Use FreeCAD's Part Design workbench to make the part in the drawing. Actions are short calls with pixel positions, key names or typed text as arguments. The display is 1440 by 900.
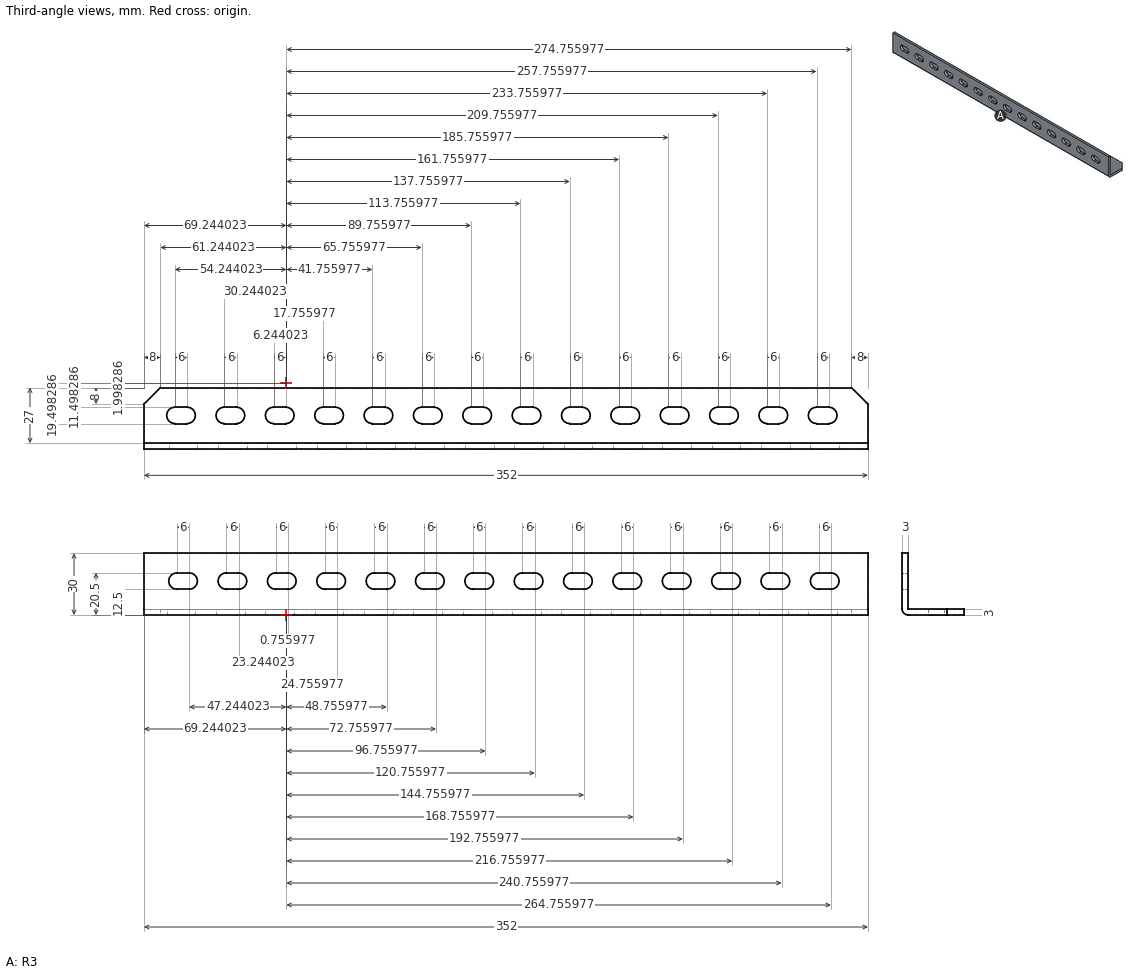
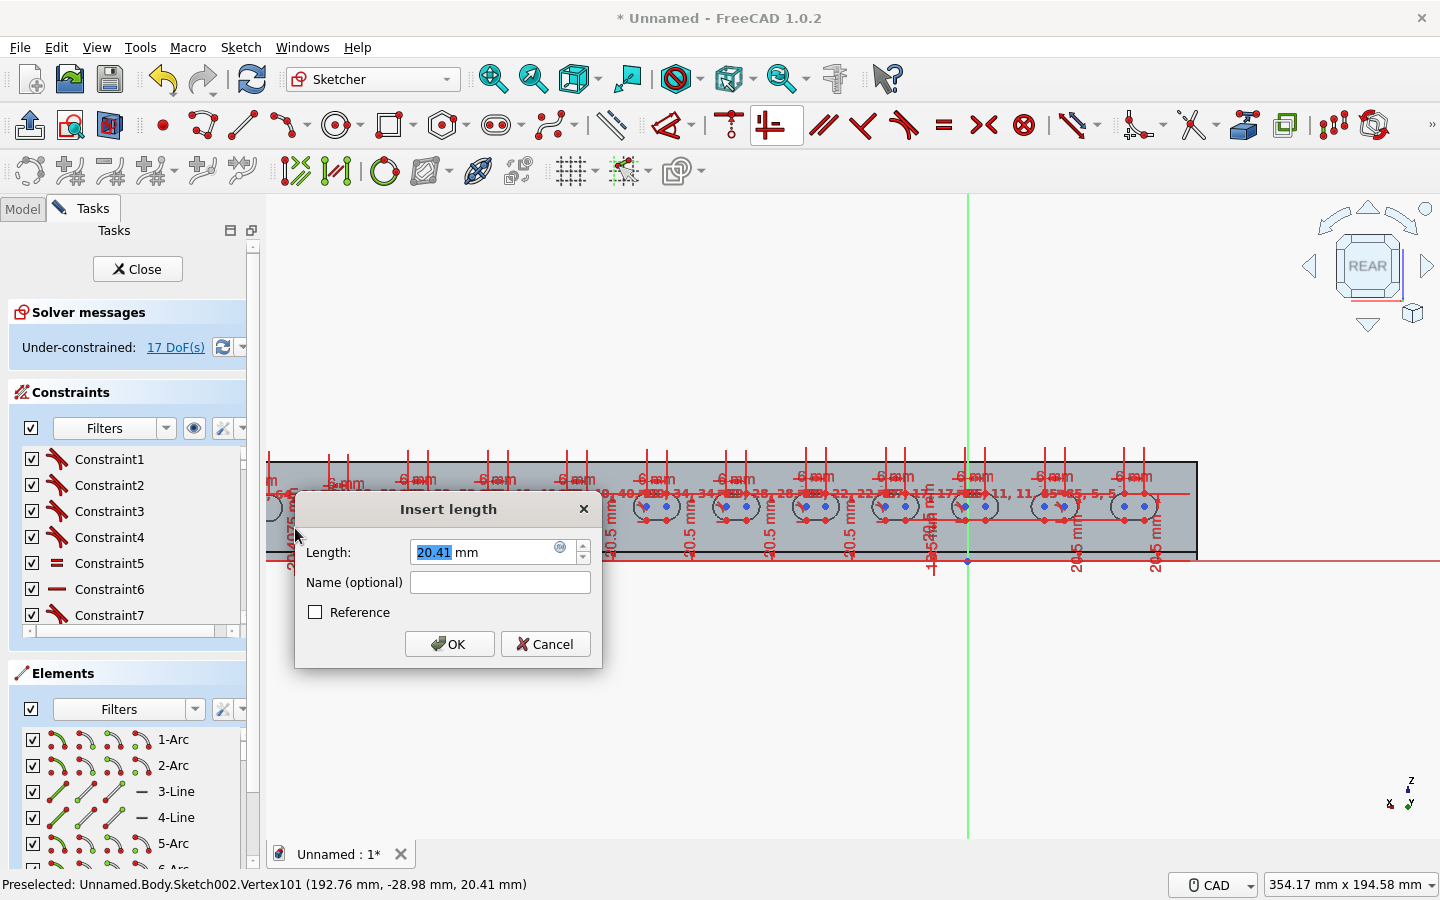
text(20.5)
key(Return)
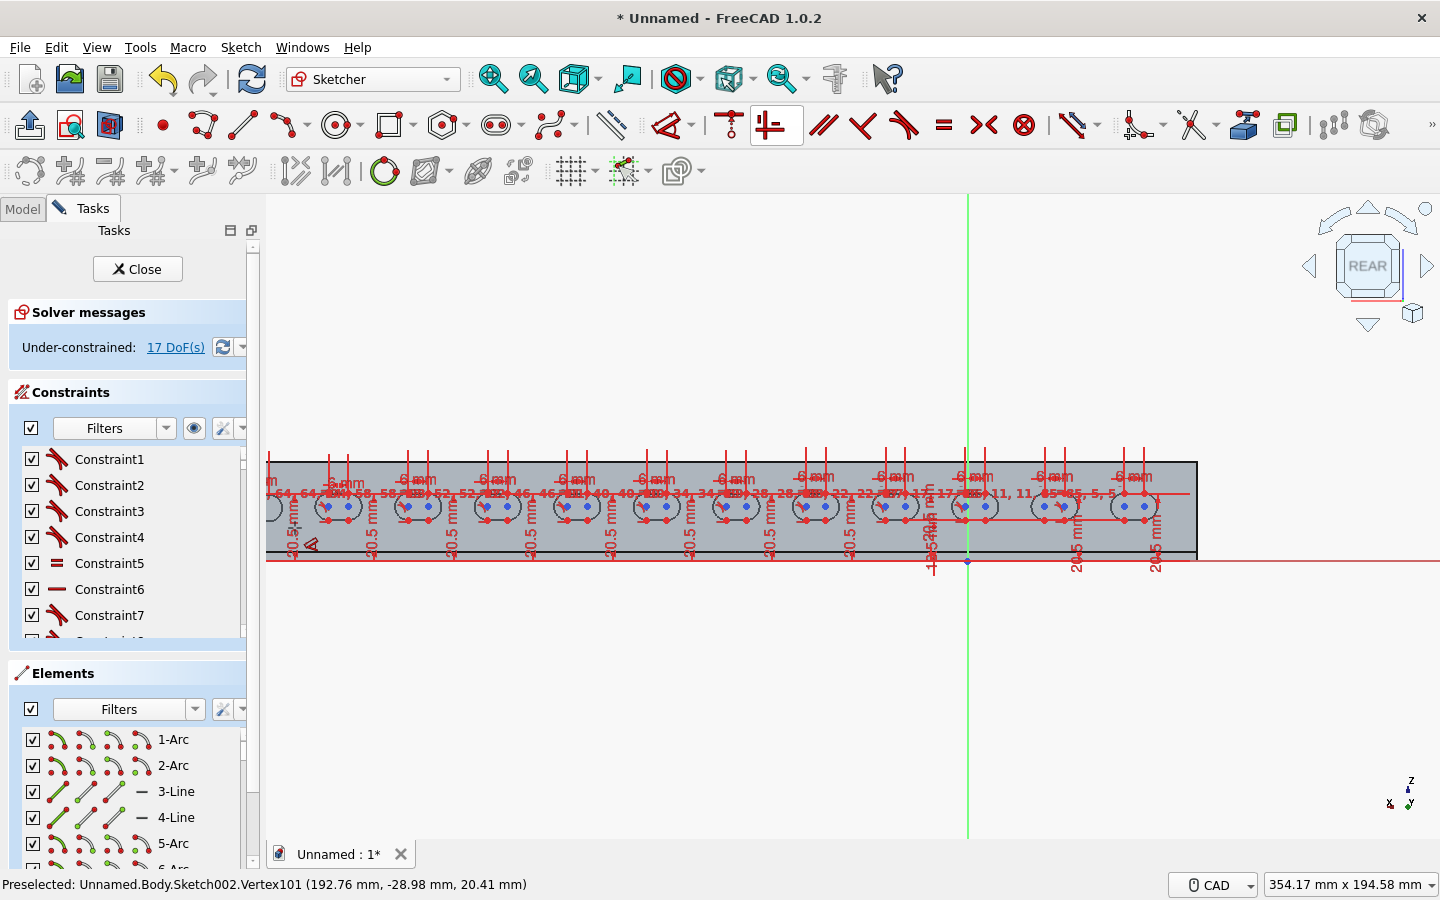
scroll(1125, 494, down, 2)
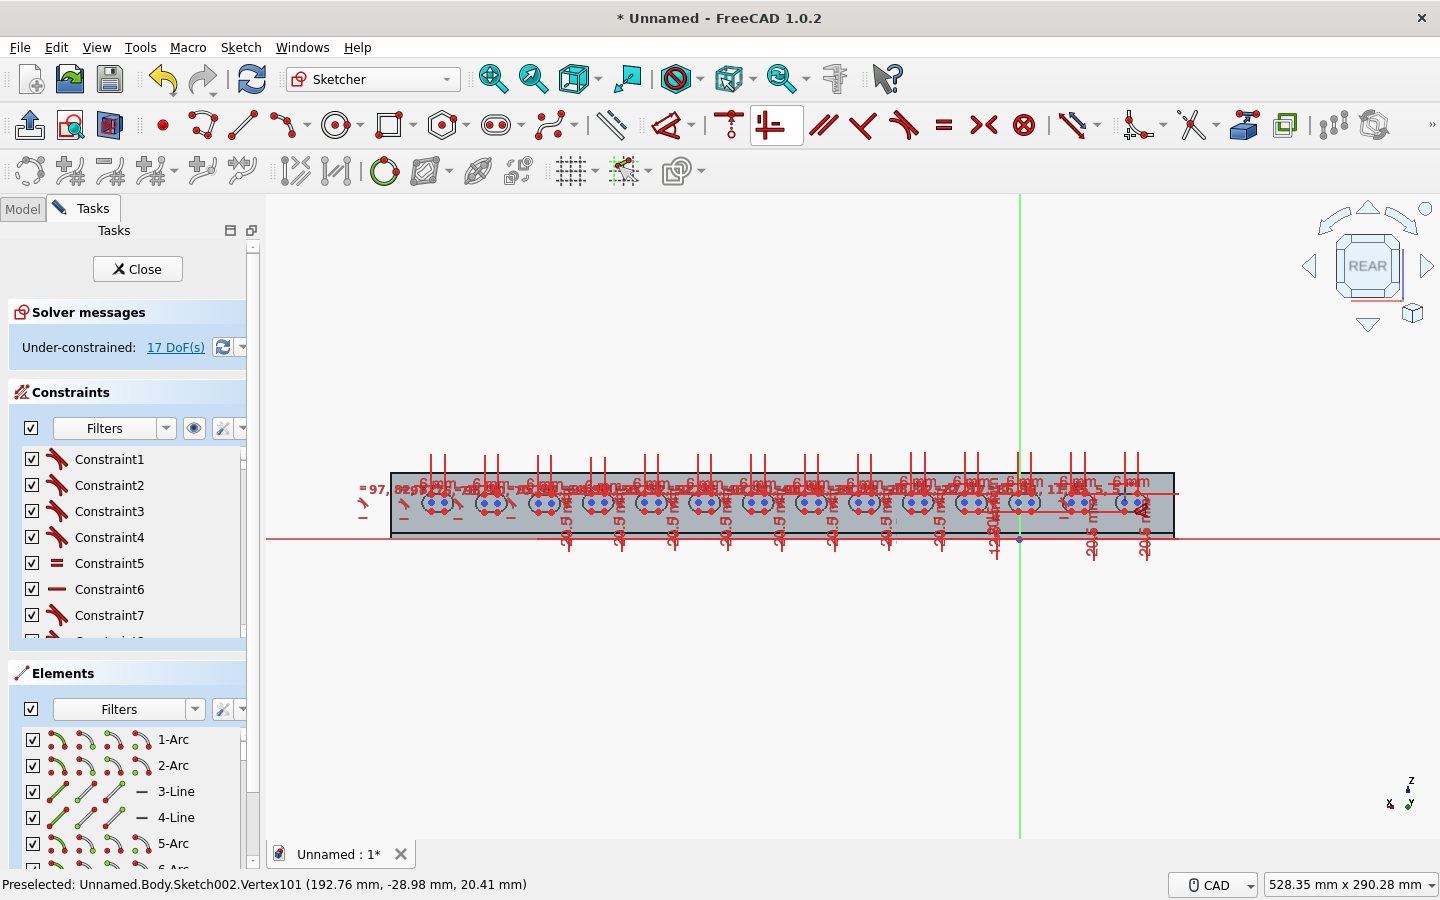
scroll(538, 495, up, 2)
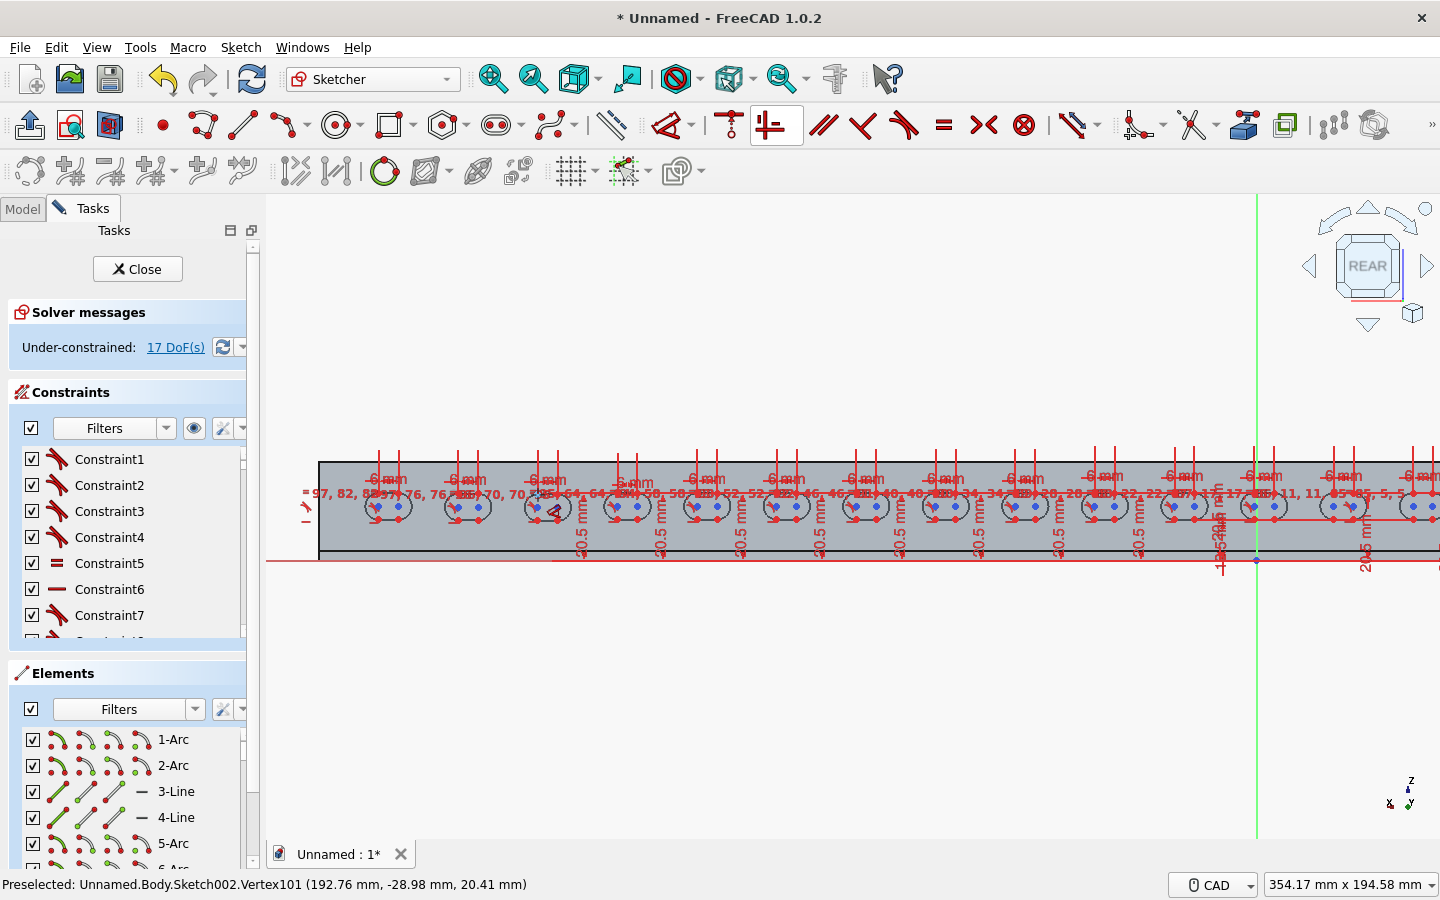
click(538, 494)
click(504, 528)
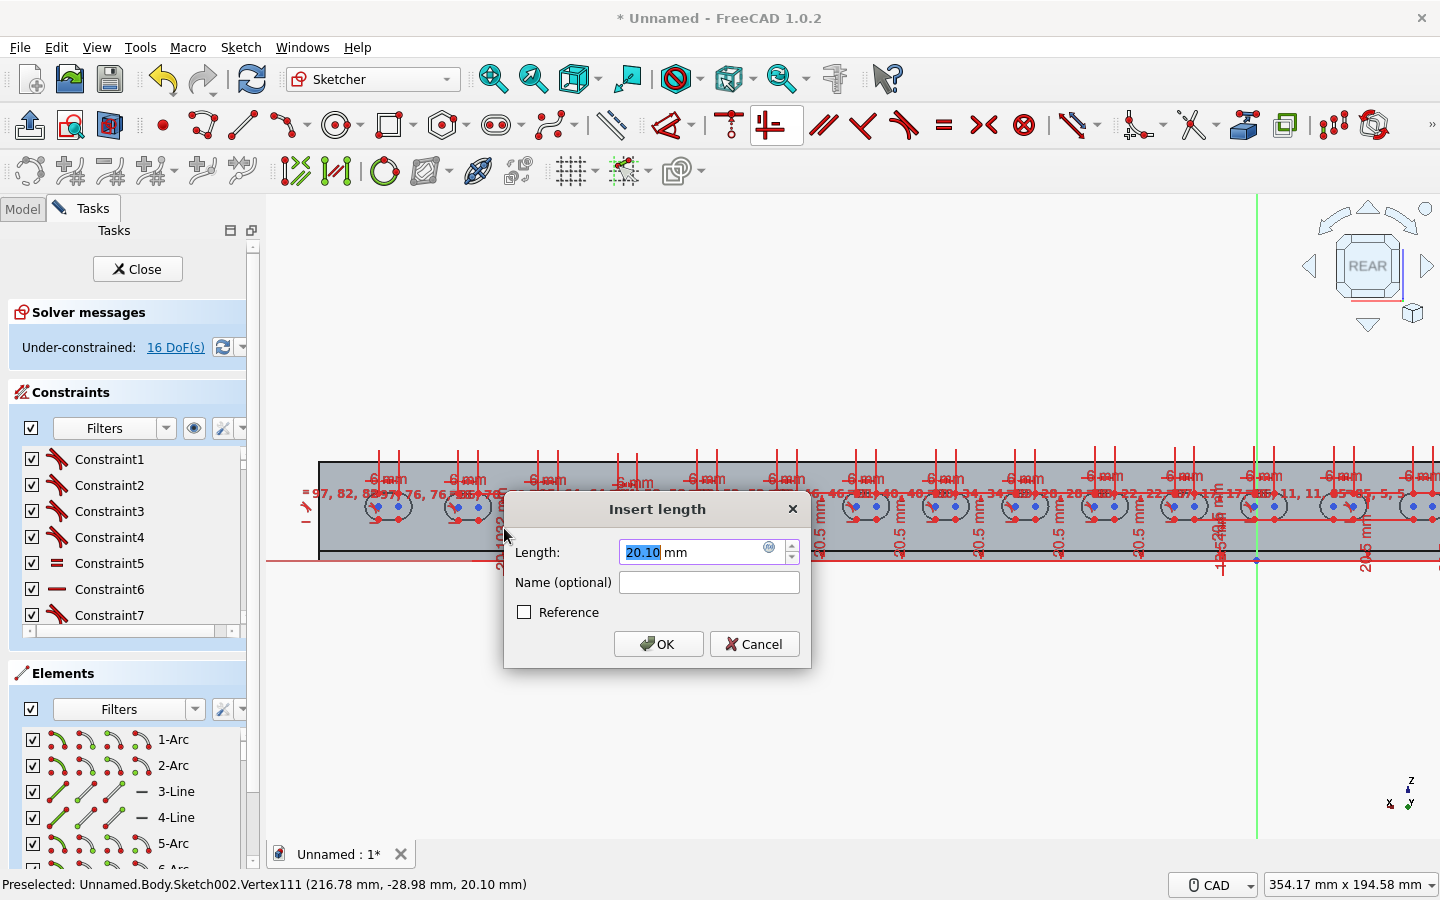
text(20.5)
key(Return)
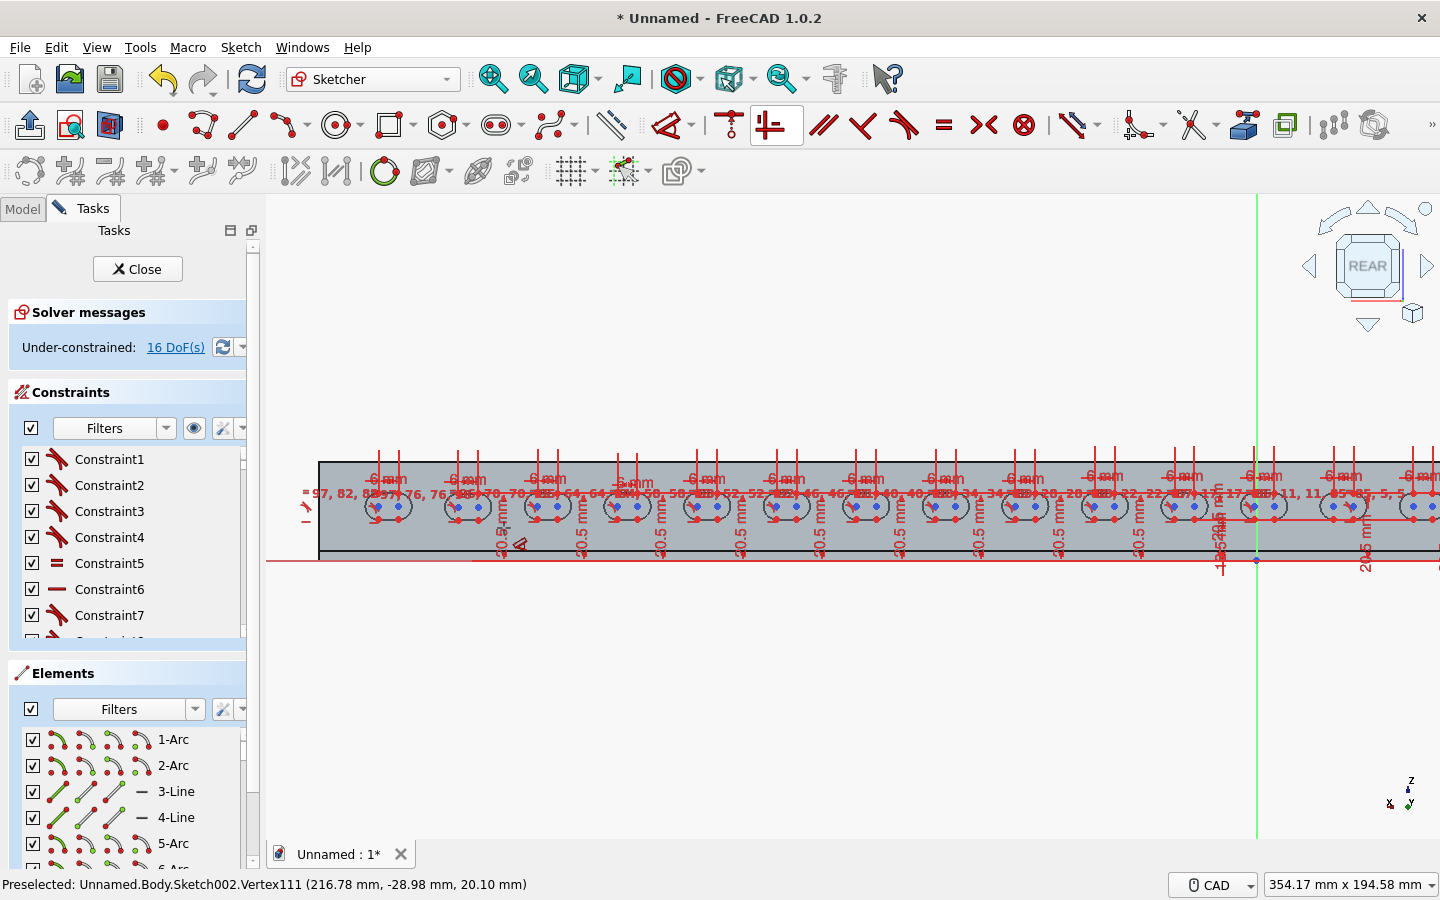
click(458, 494)
click(424, 527)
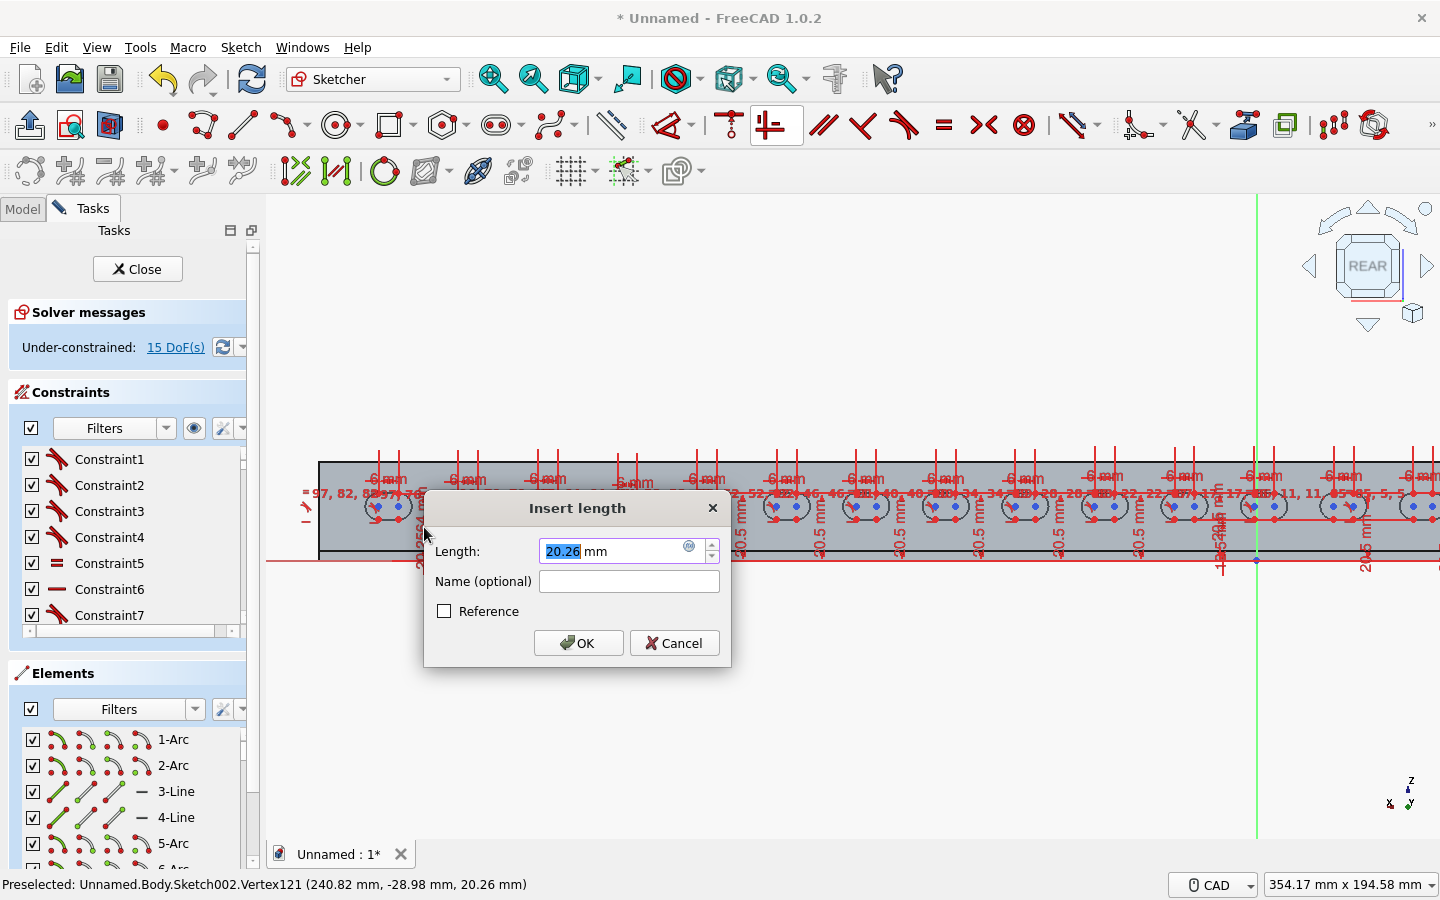
text(20.5)
key(Return)